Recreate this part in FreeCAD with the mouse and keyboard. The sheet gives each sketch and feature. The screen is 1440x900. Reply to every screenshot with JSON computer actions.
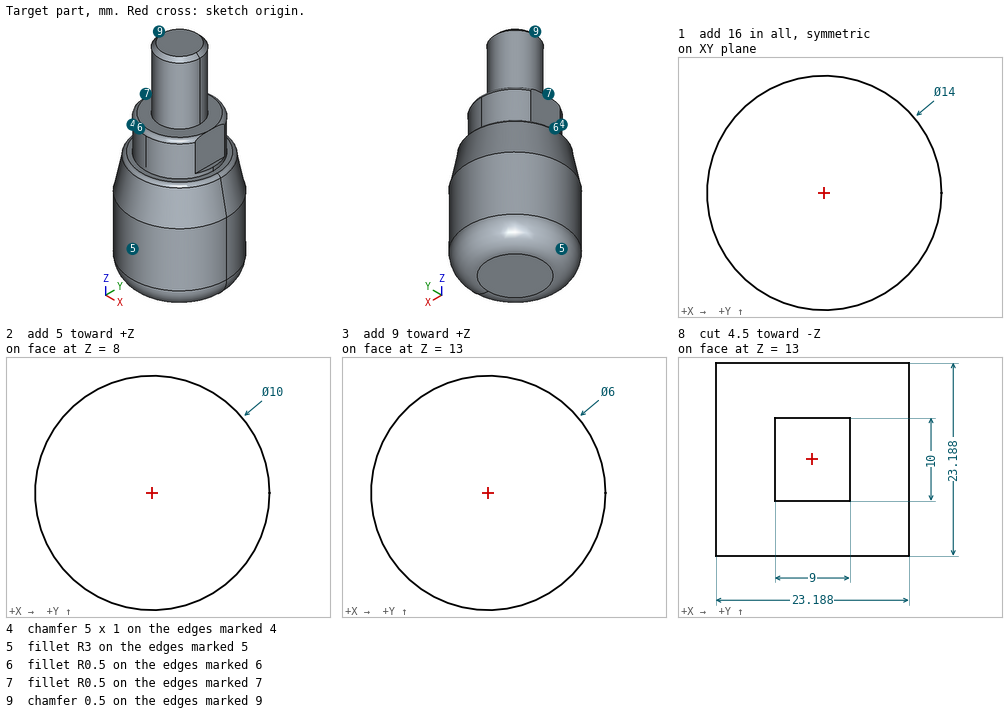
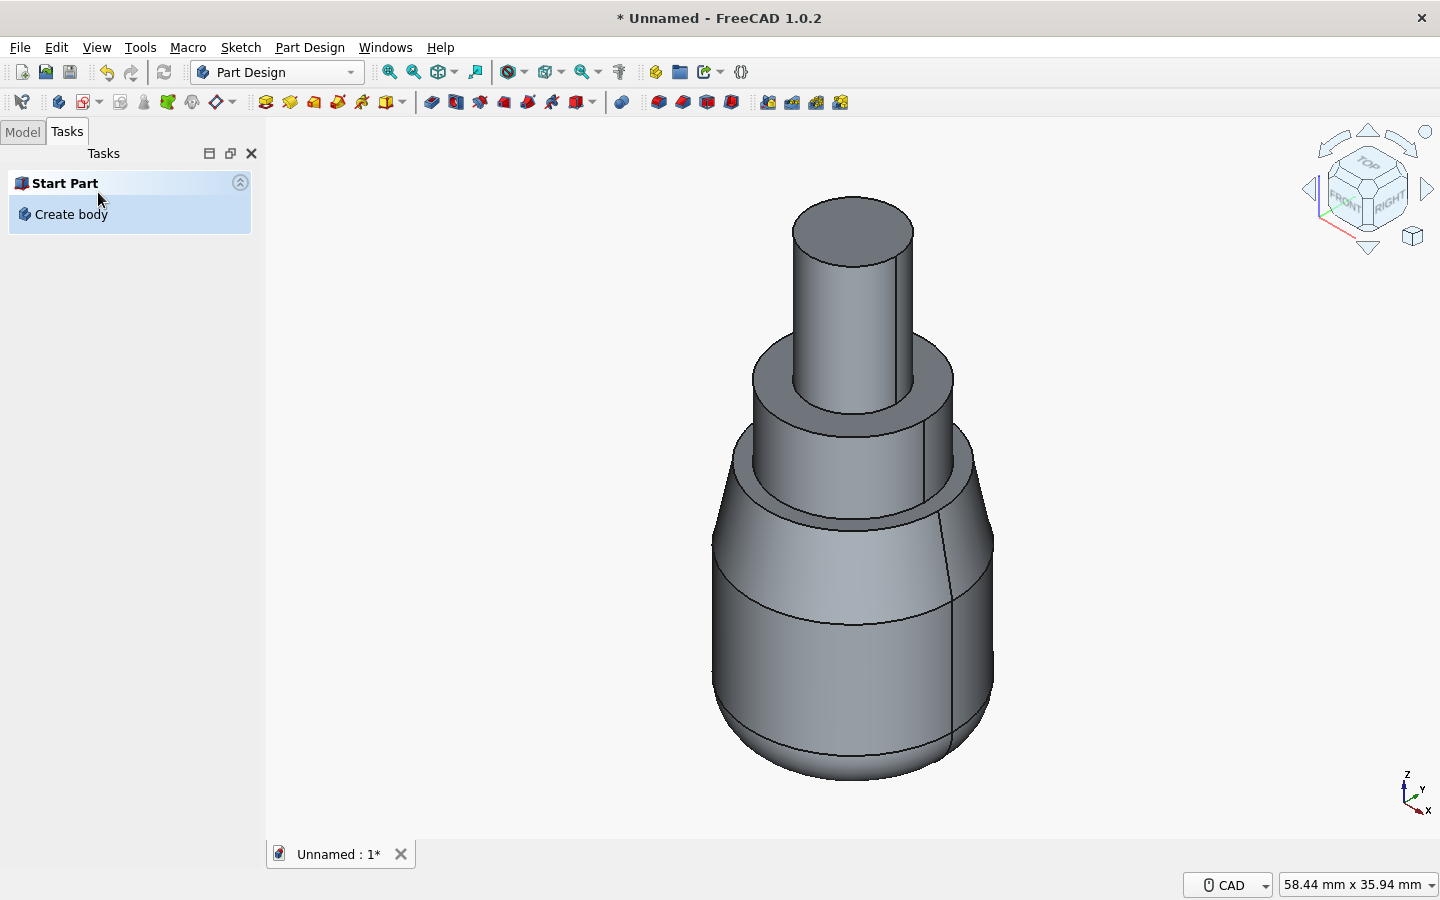
{"action": "key", "text": "v f"}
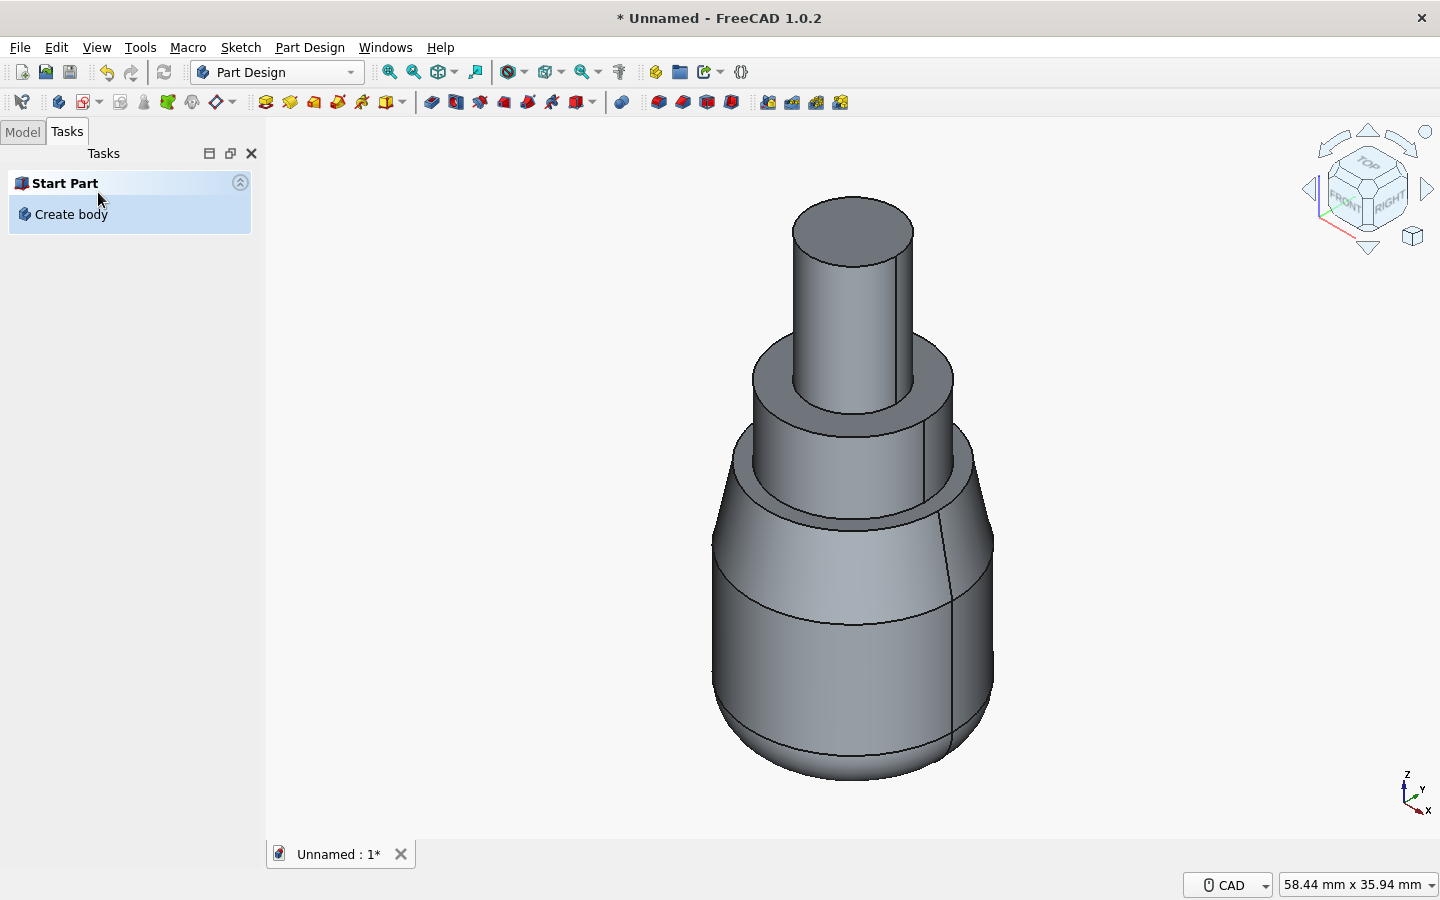
{"action": "left_click", "coordinate": [746, 492]}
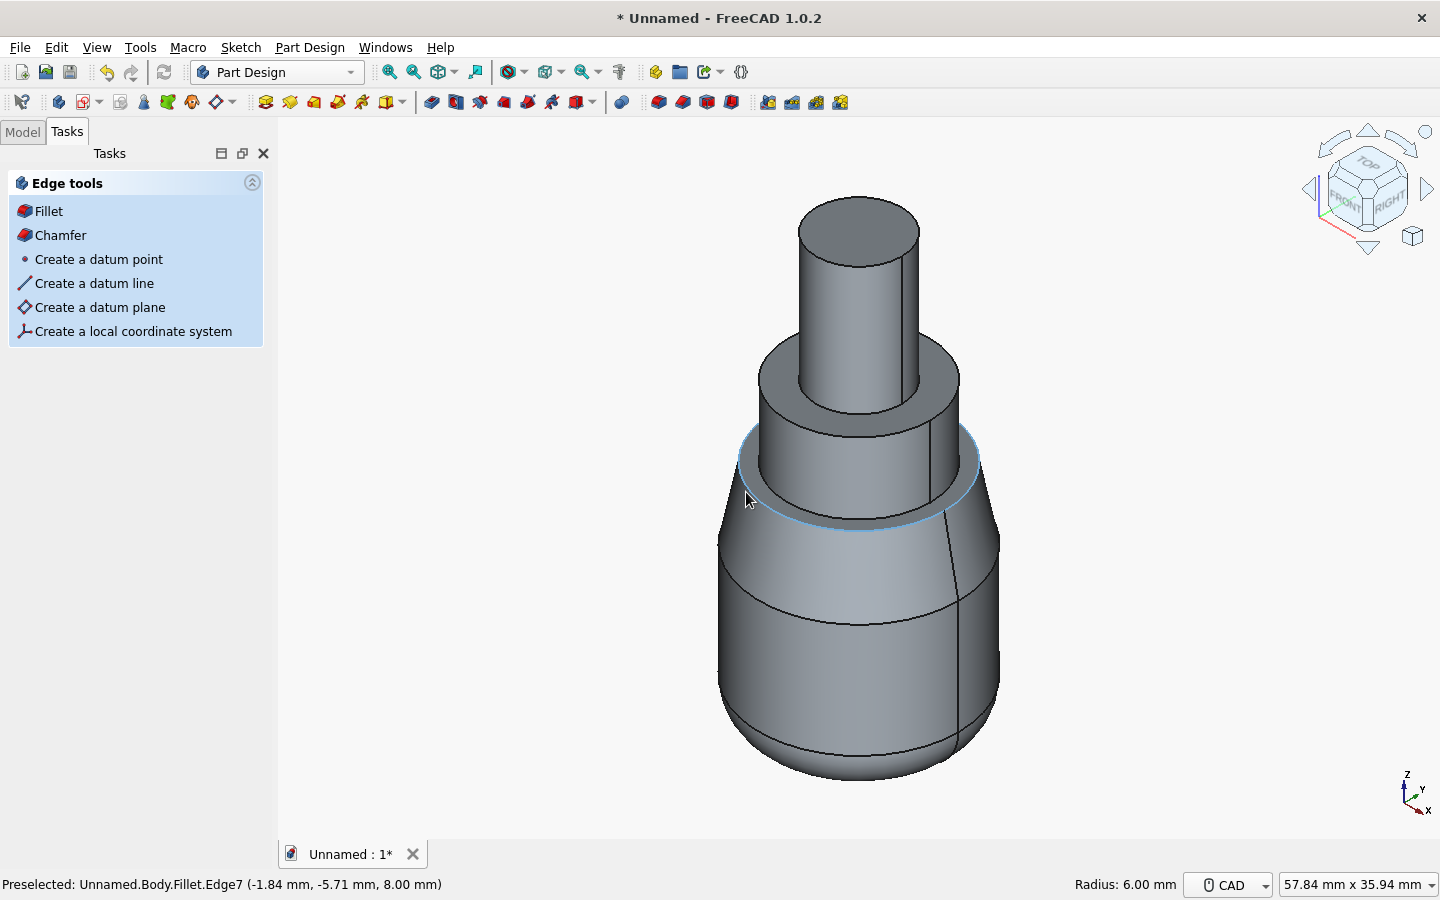
{"action": "left_click", "coordinate": [660, 102]}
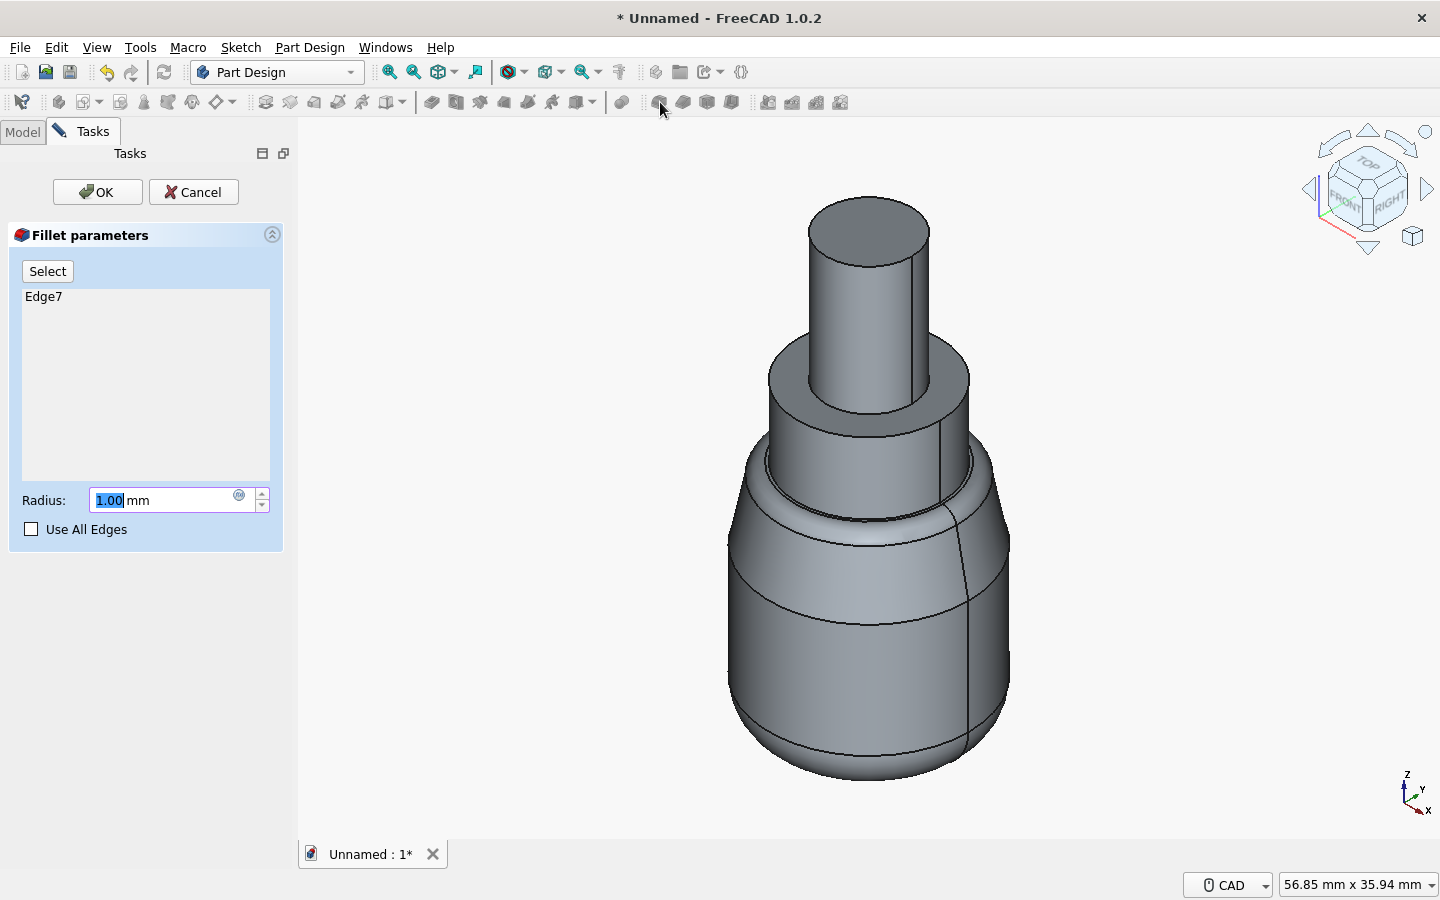
{"action": "type", "text": "0.5"}
{"action": "key", "text": "Tab"}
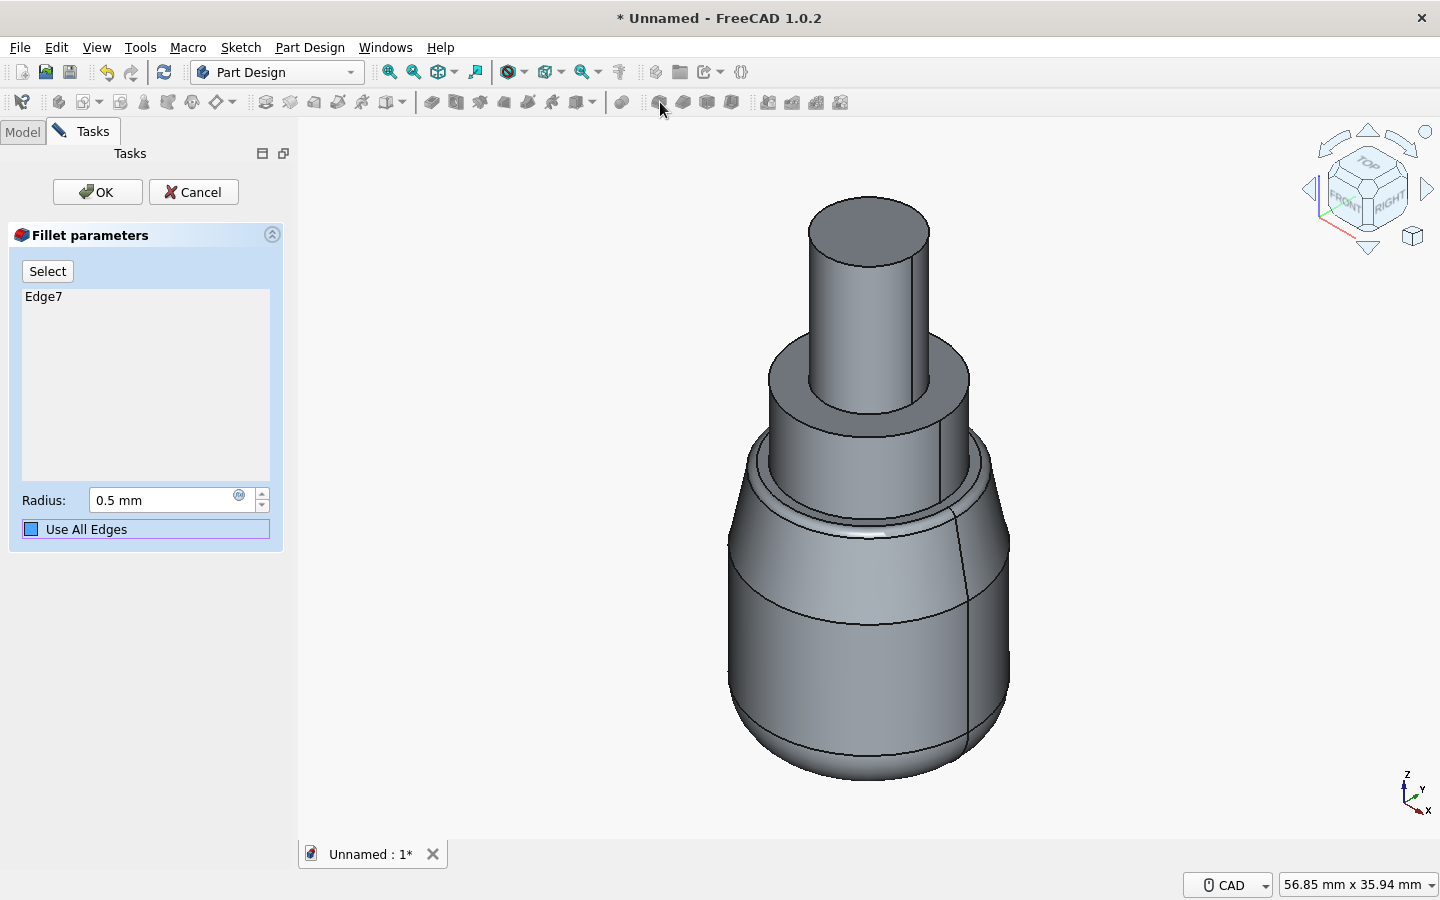
{"action": "left_click", "coordinate": [98, 192]}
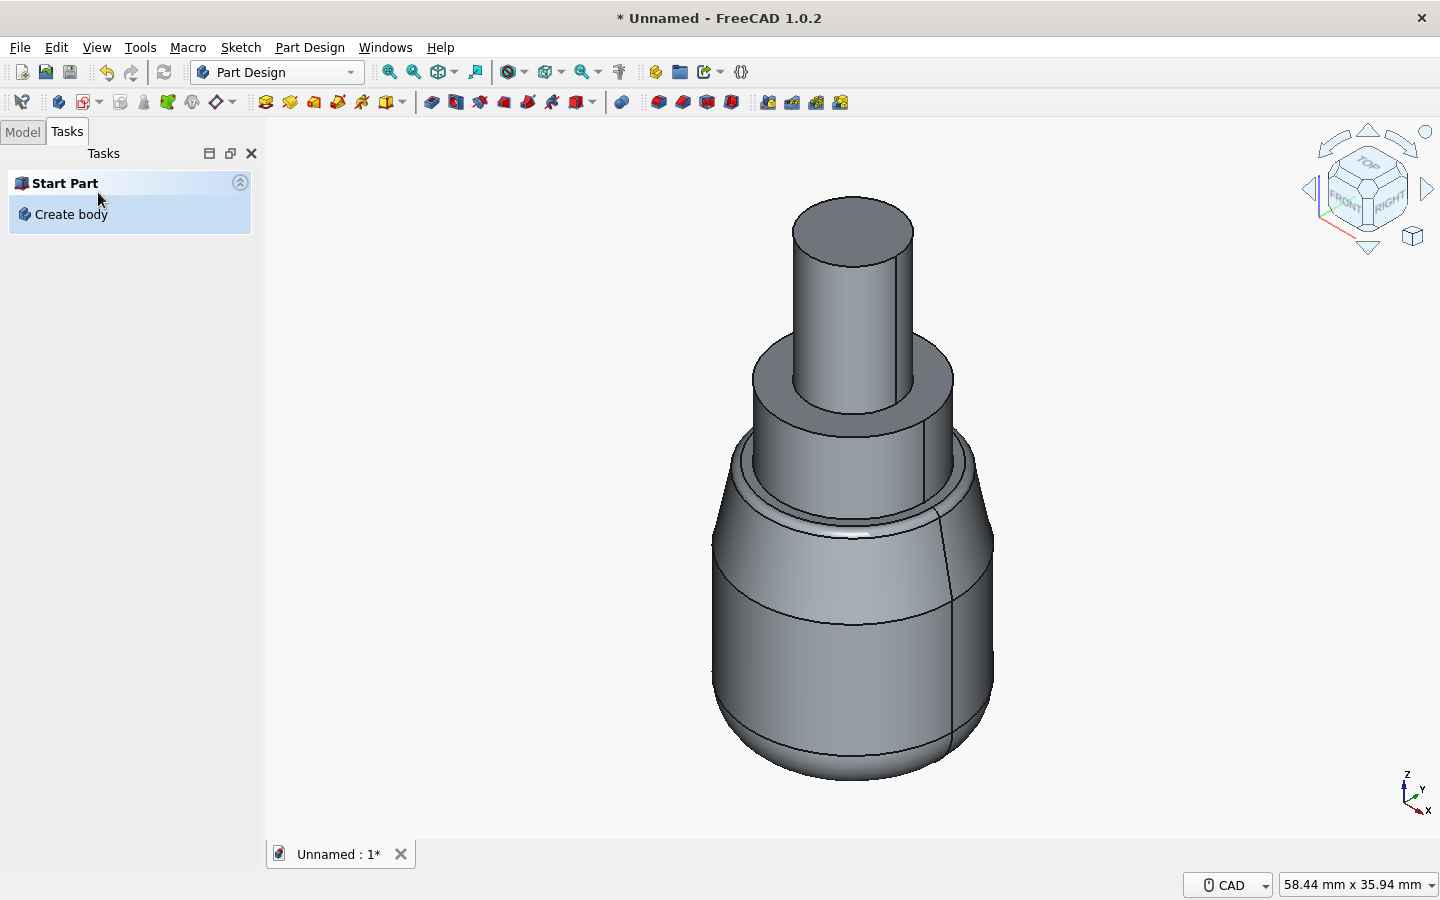
{"action": "key", "text": "v f"}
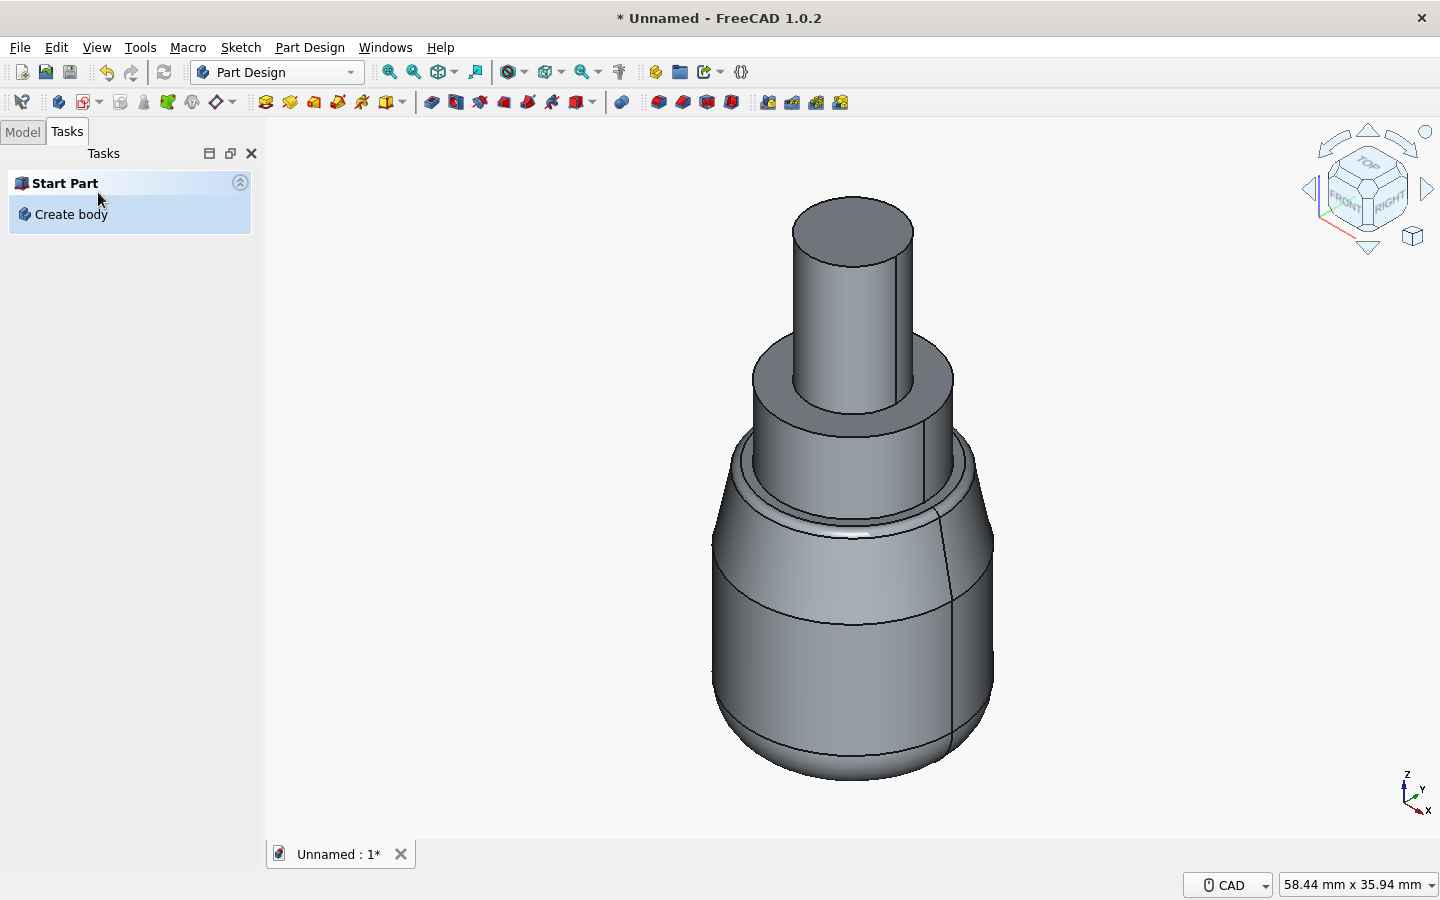
{"action": "left_click", "coordinate": [764, 405]}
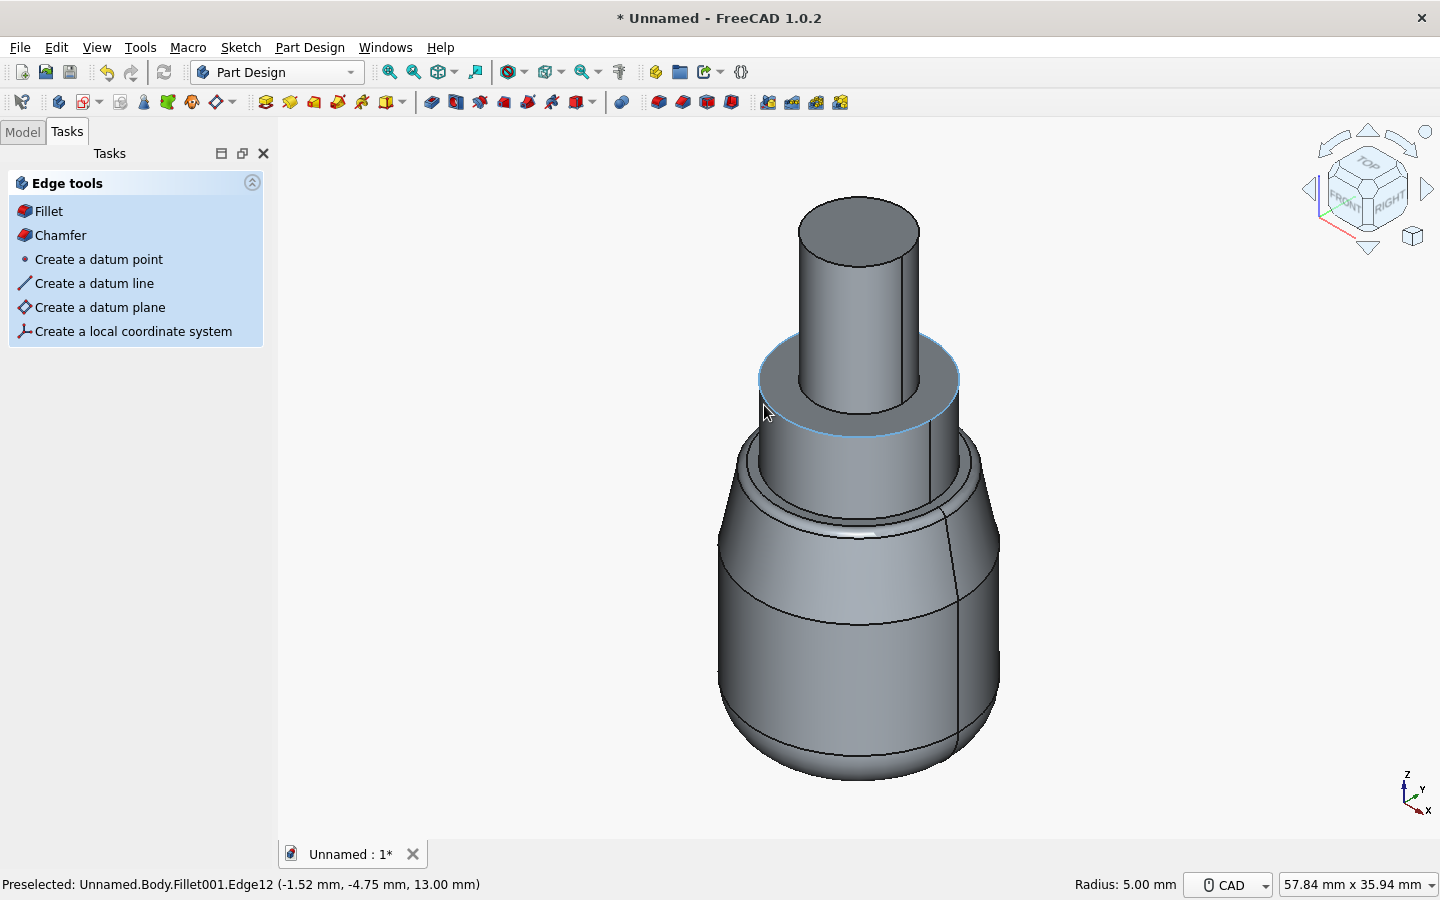
{"action": "left_click", "coordinate": [660, 102]}